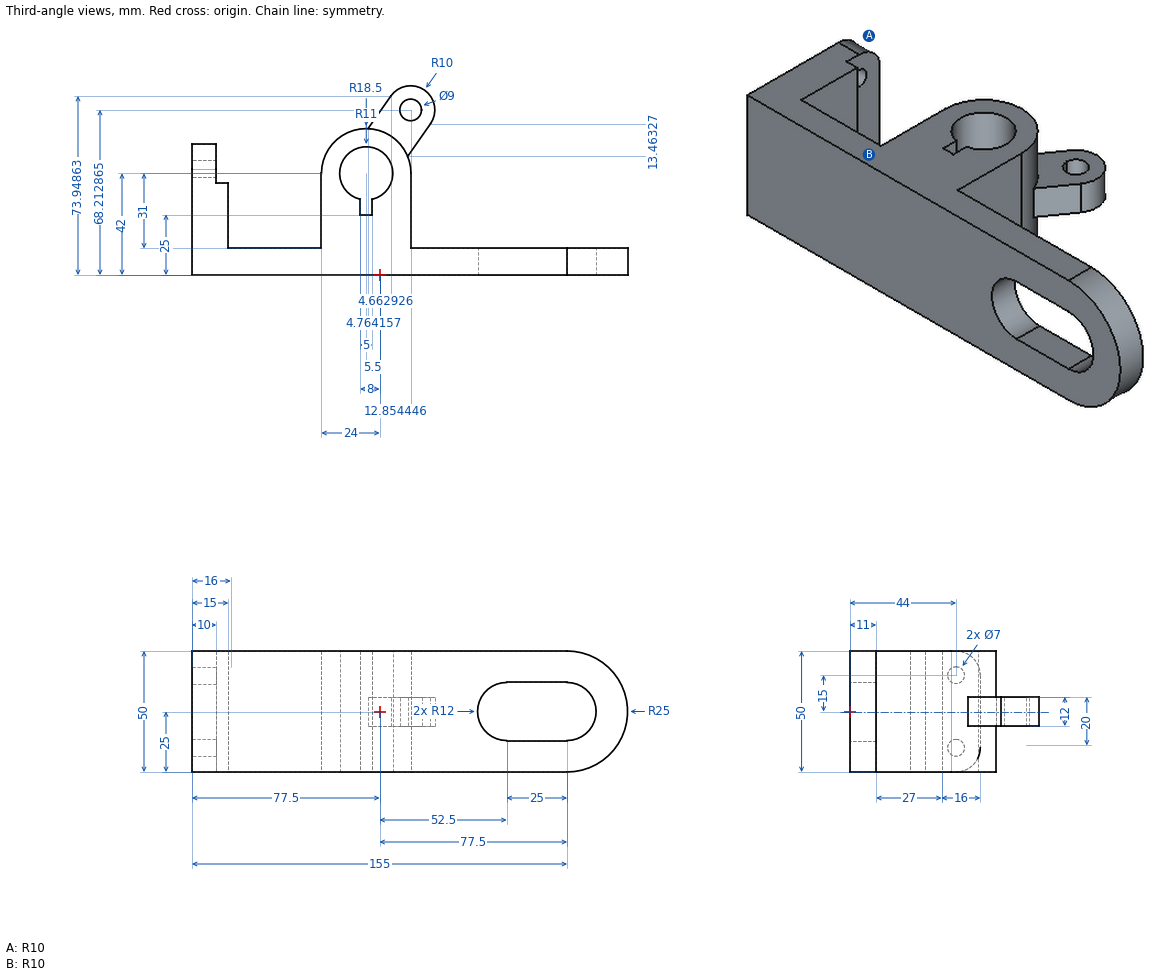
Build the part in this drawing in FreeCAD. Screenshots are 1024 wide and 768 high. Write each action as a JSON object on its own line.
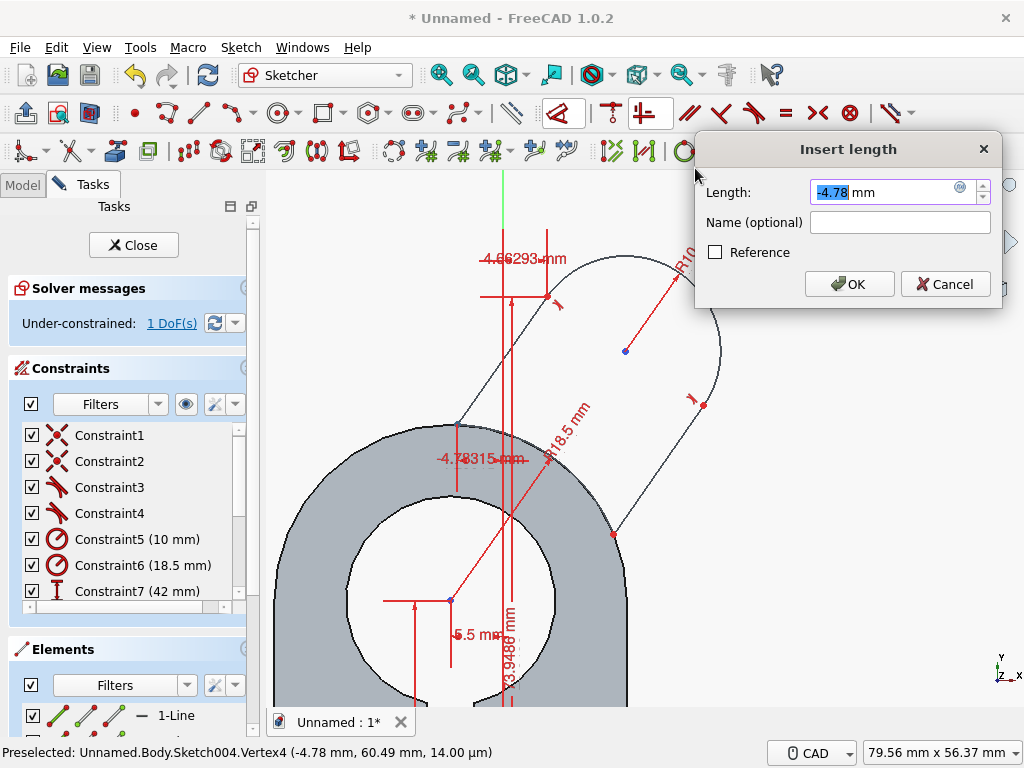
{"action": "type", "text": "-4.764157"}
{"action": "key", "text": "Return"}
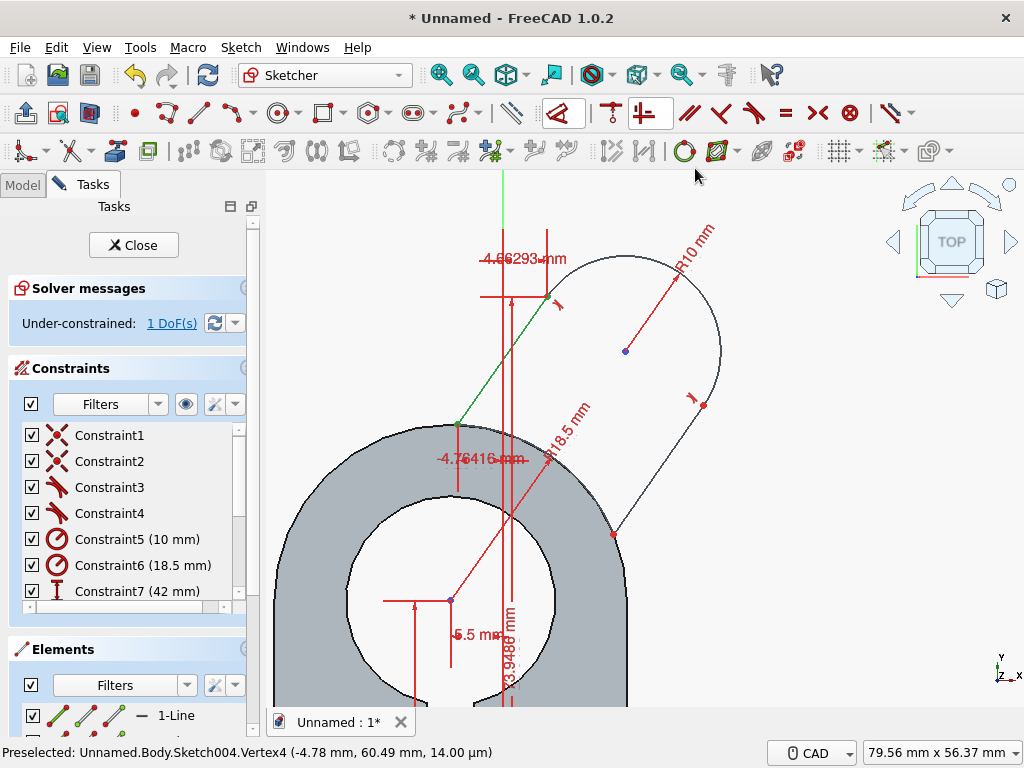
{"action": "left_click", "coordinate": [641, 496]}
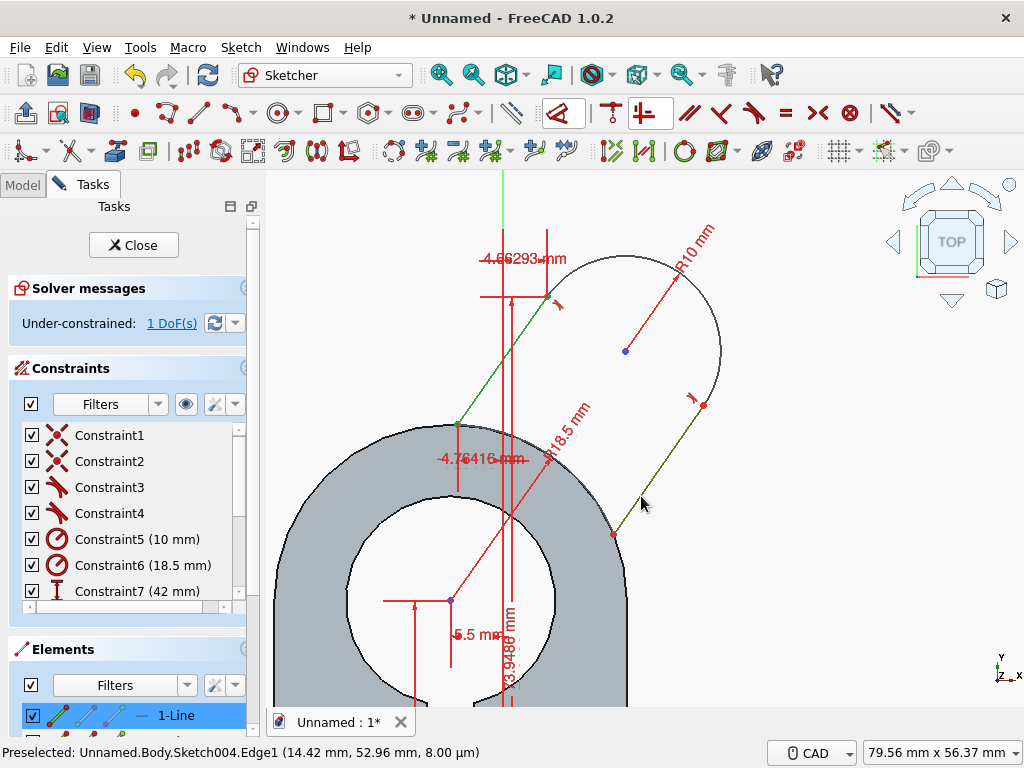
{"action": "left_click", "coordinate": [580, 114]}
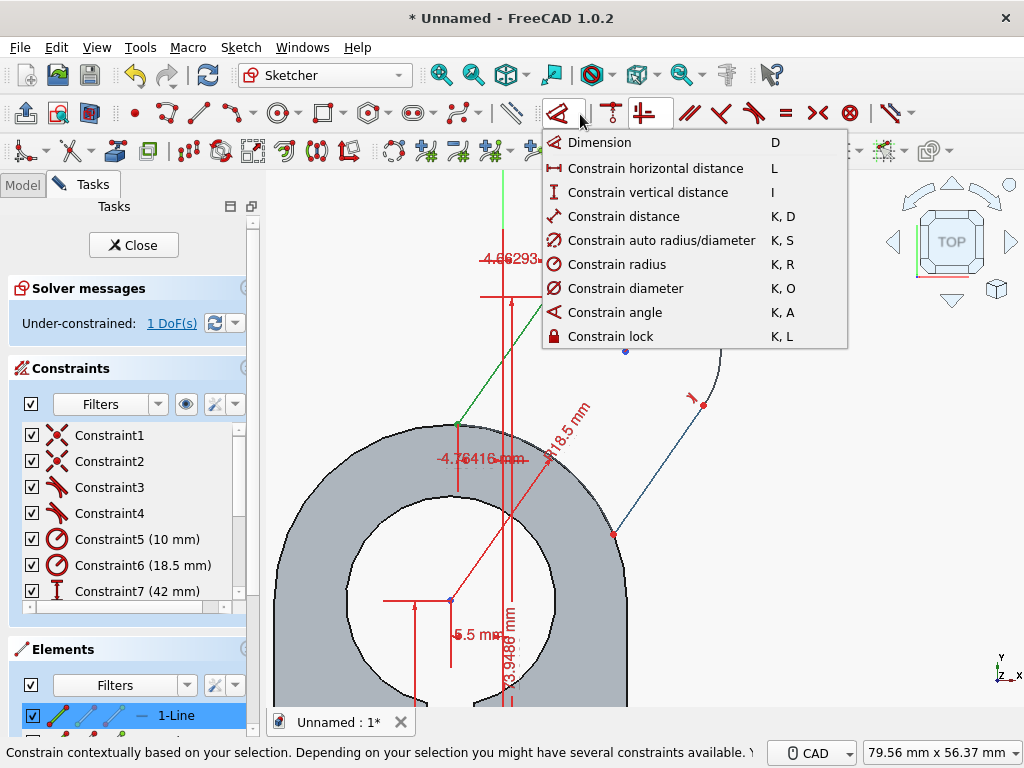
{"action": "left_click", "coordinate": [695, 192]}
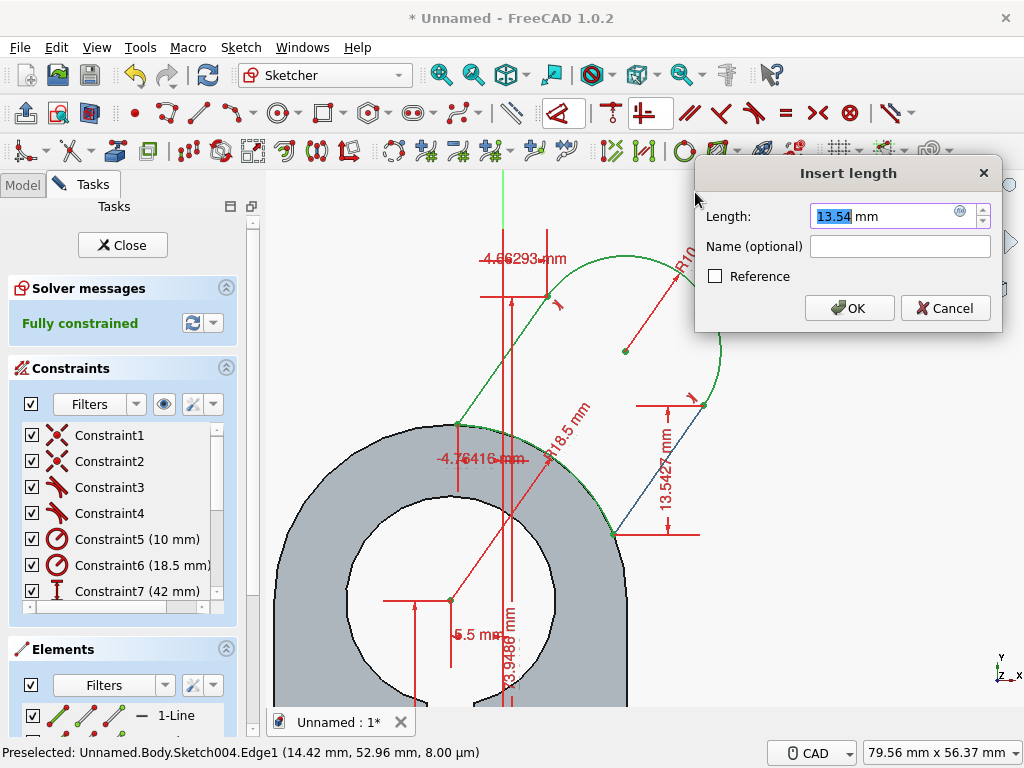
{"action": "type", "text": "13.46327"}
{"action": "key", "text": "Return"}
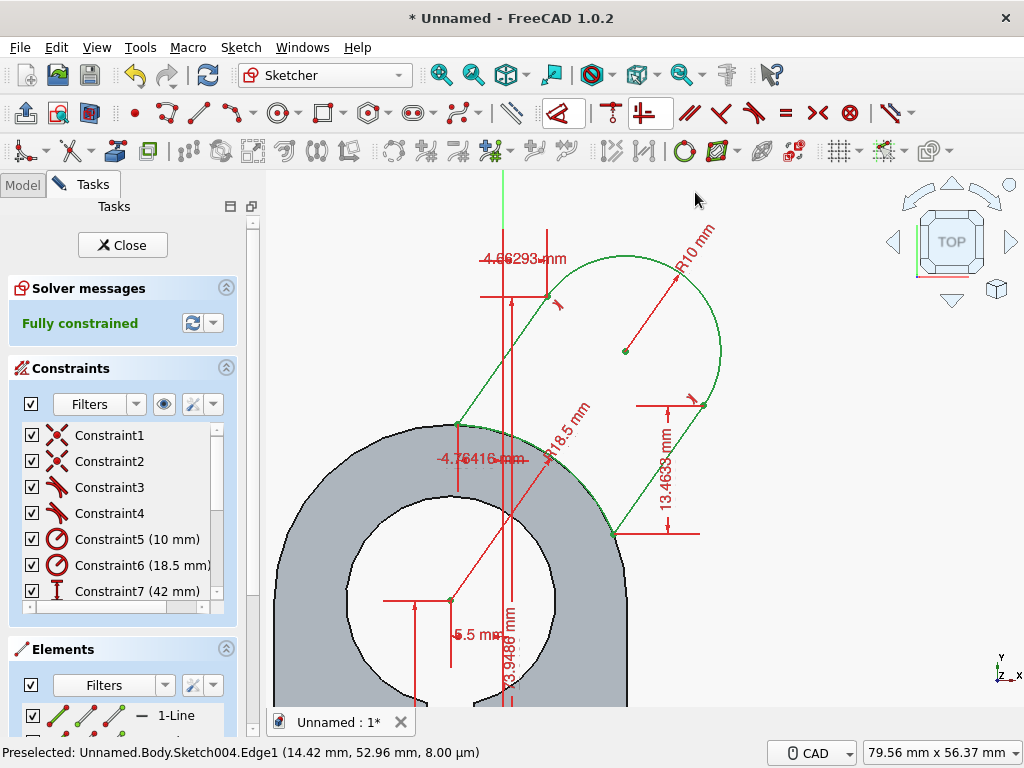
{"action": "left_click", "coordinate": [123, 245]}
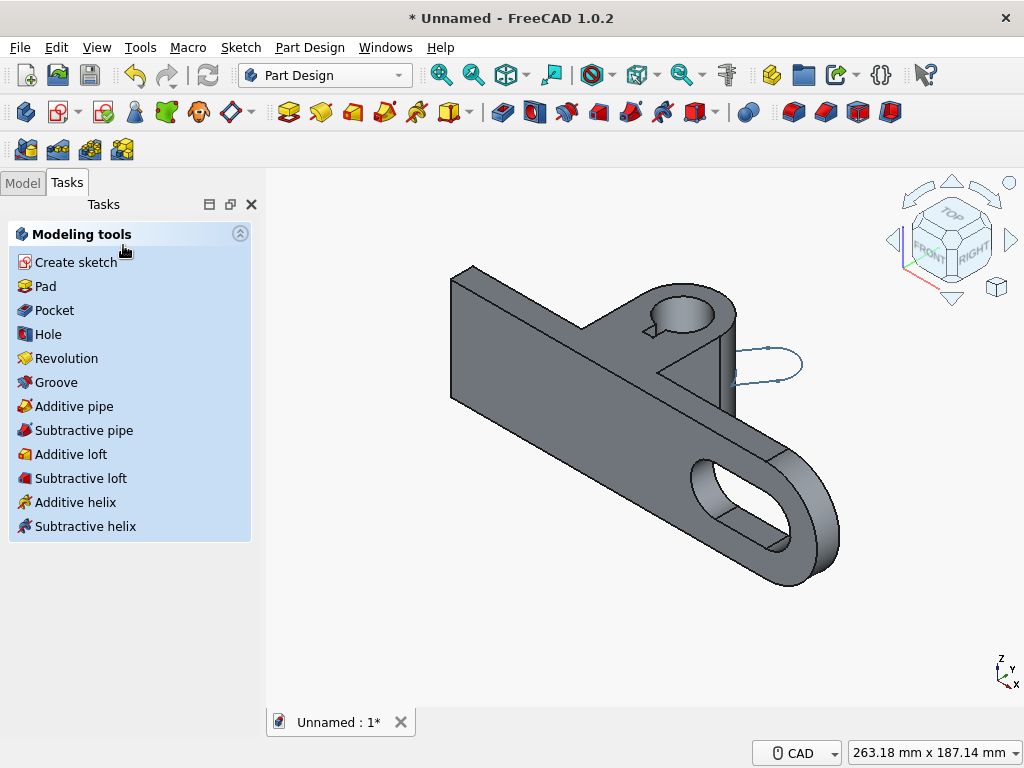
{"action": "left_click", "coordinate": [290, 112]}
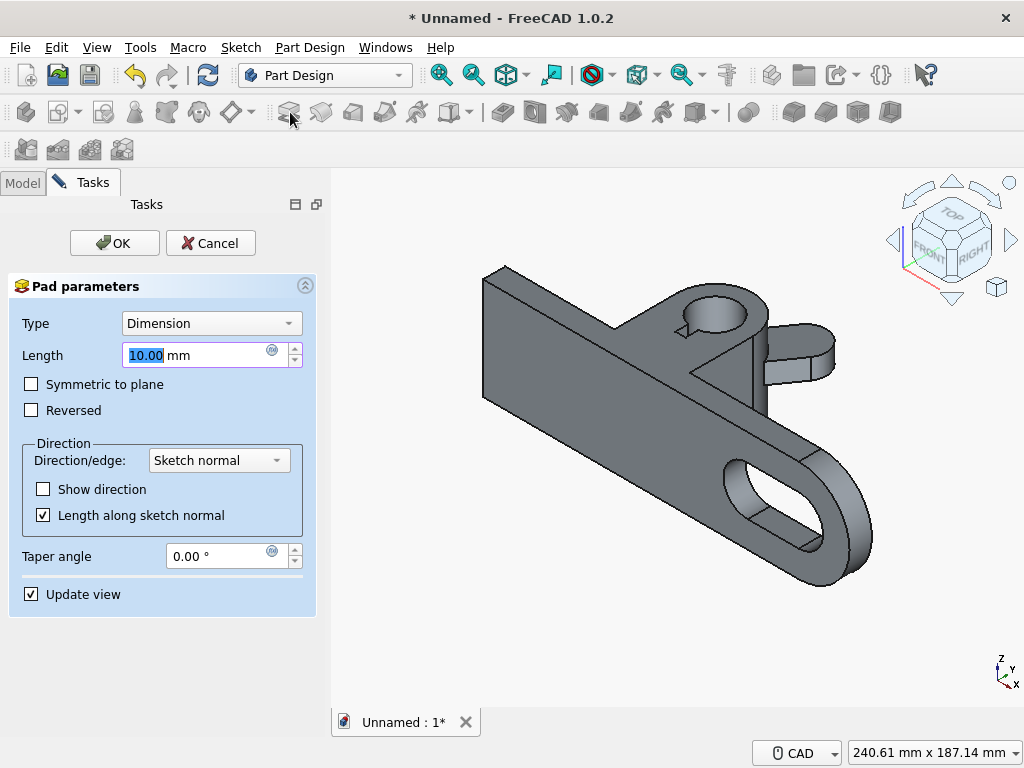
{"action": "type", "text": "12"}
{"action": "key", "text": "Tab"}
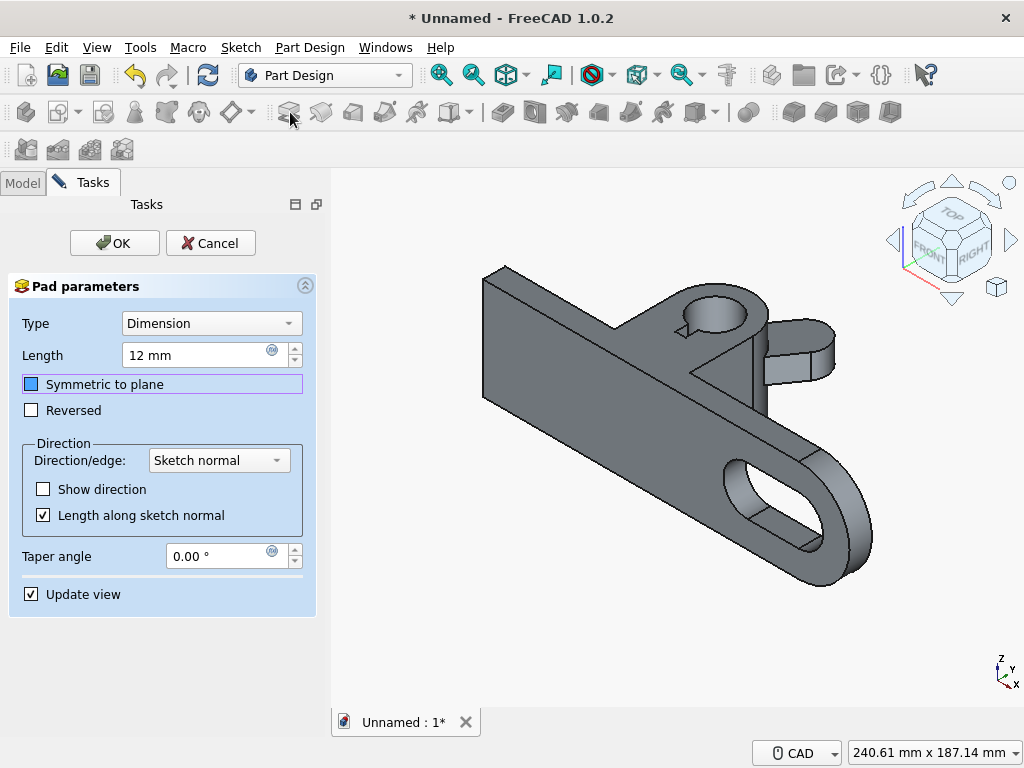
{"action": "left_click", "coordinate": [30, 384]}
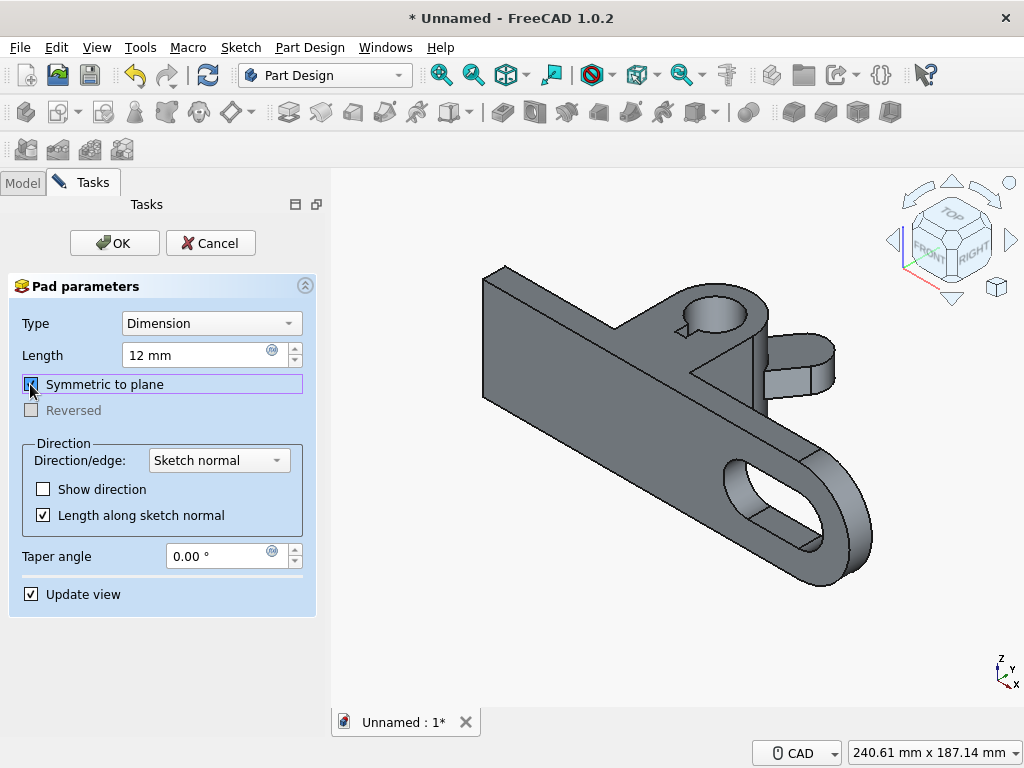
{"action": "left_click", "coordinate": [115, 243]}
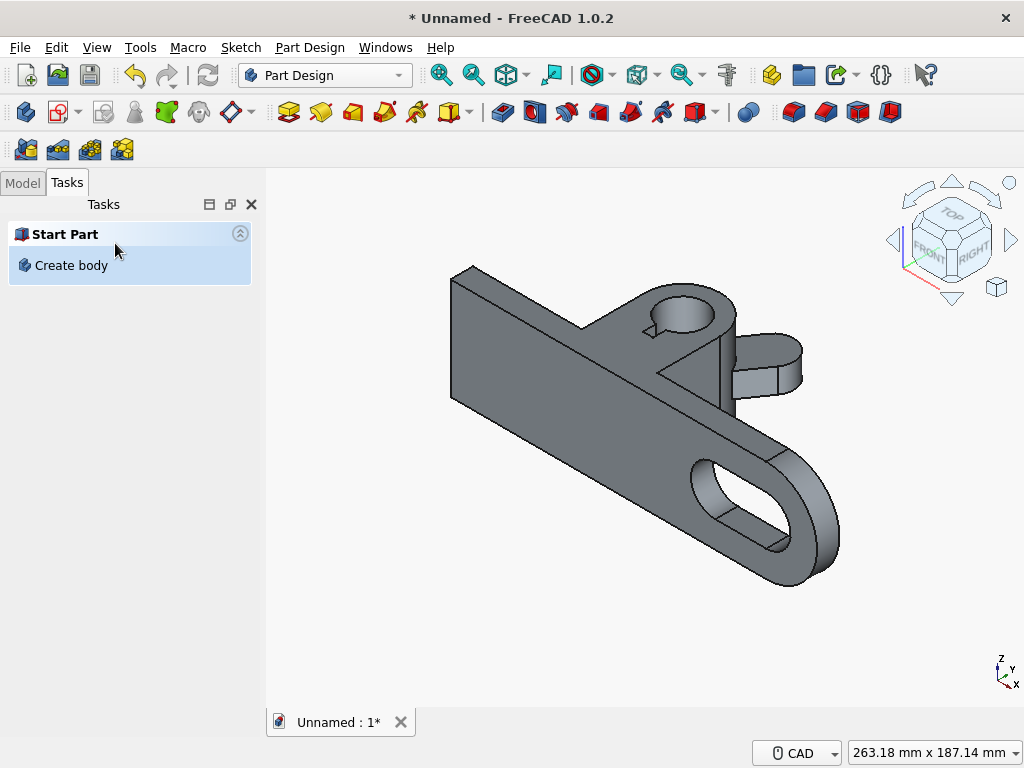
{"action": "left_click", "coordinate": [773, 350]}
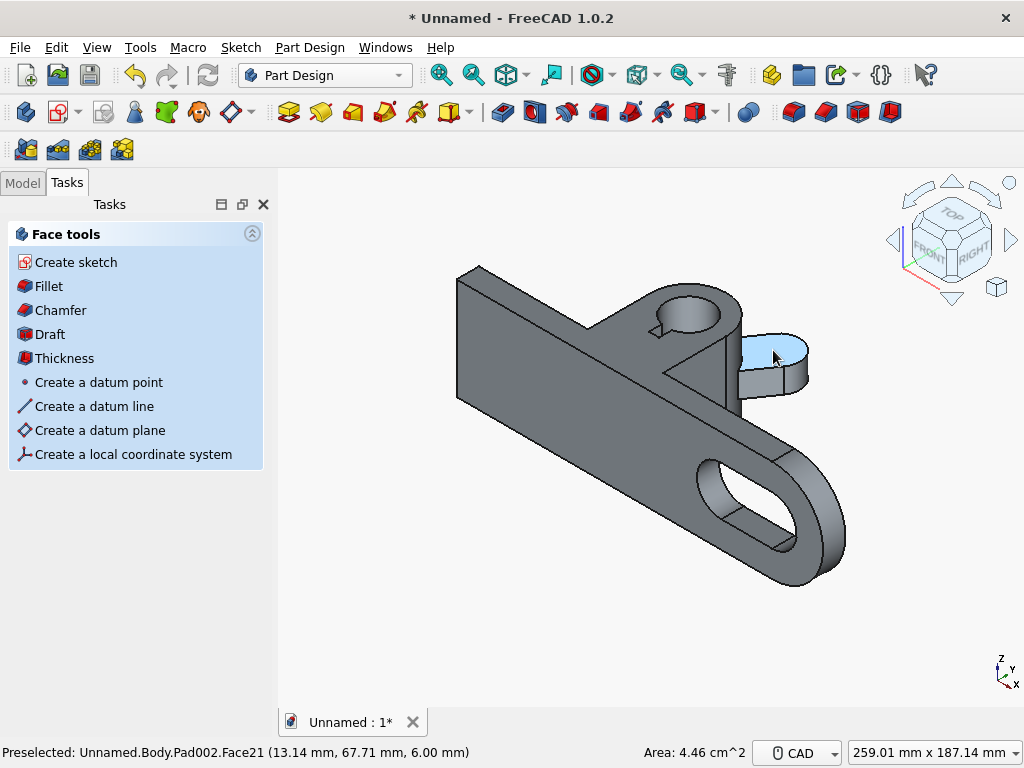
{"action": "left_click", "coordinate": [58, 112]}